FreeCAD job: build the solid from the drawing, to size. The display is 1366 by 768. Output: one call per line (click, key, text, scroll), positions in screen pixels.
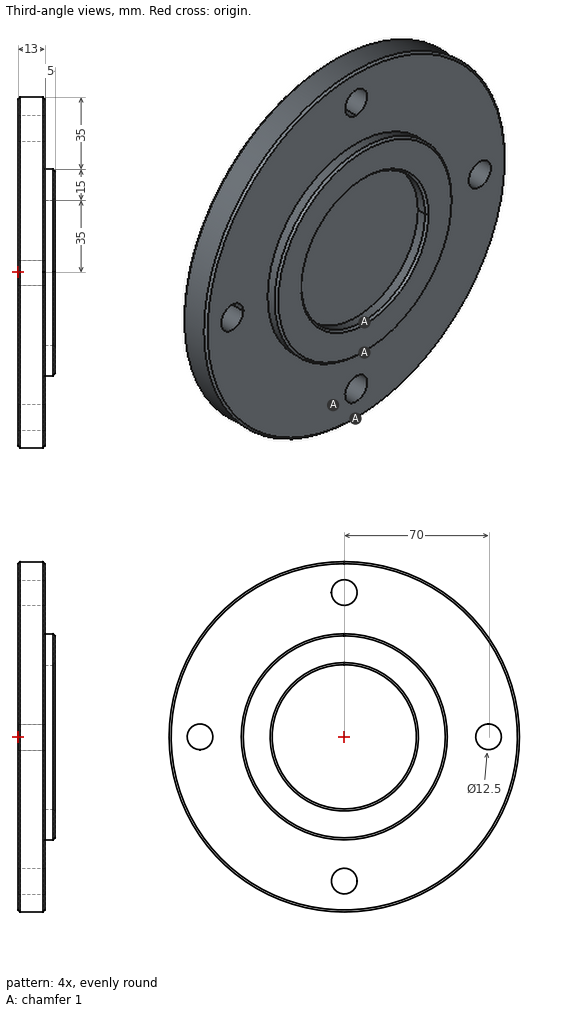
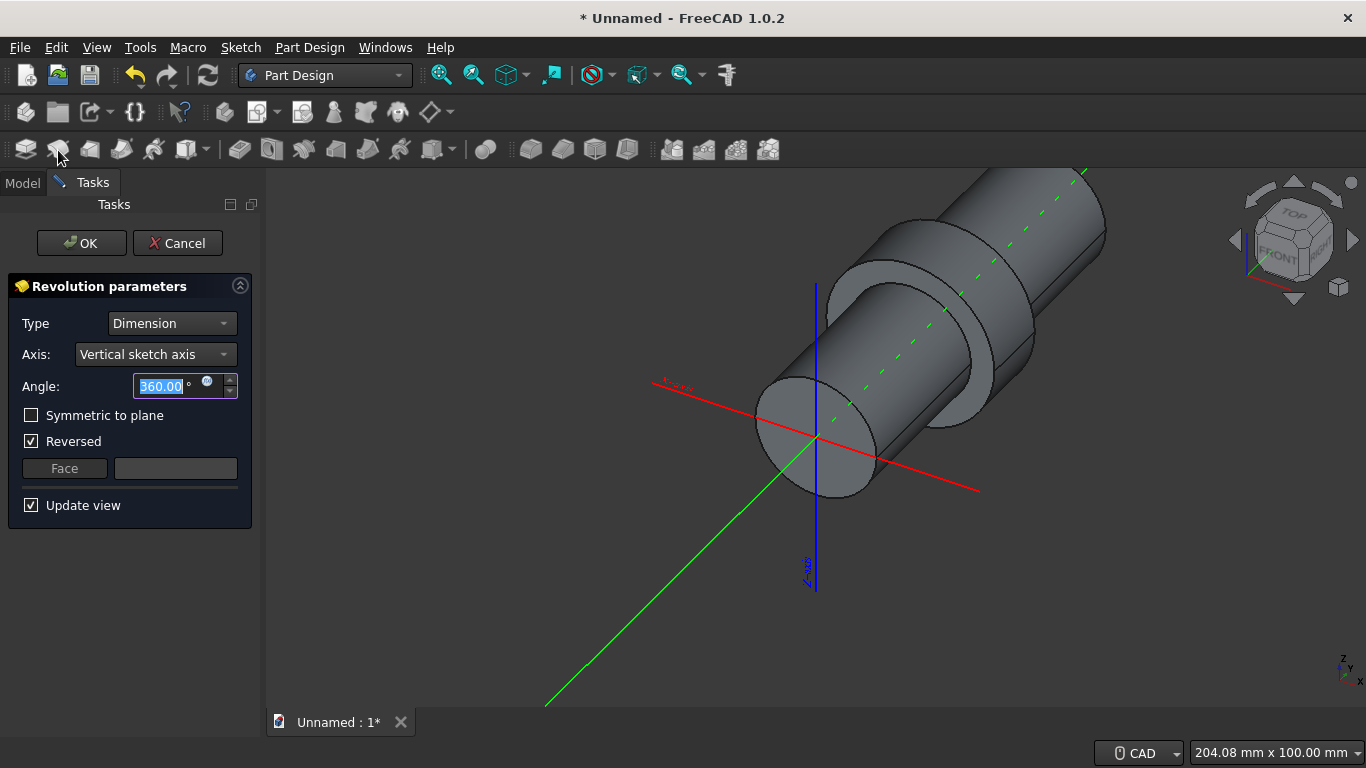
click(156, 354)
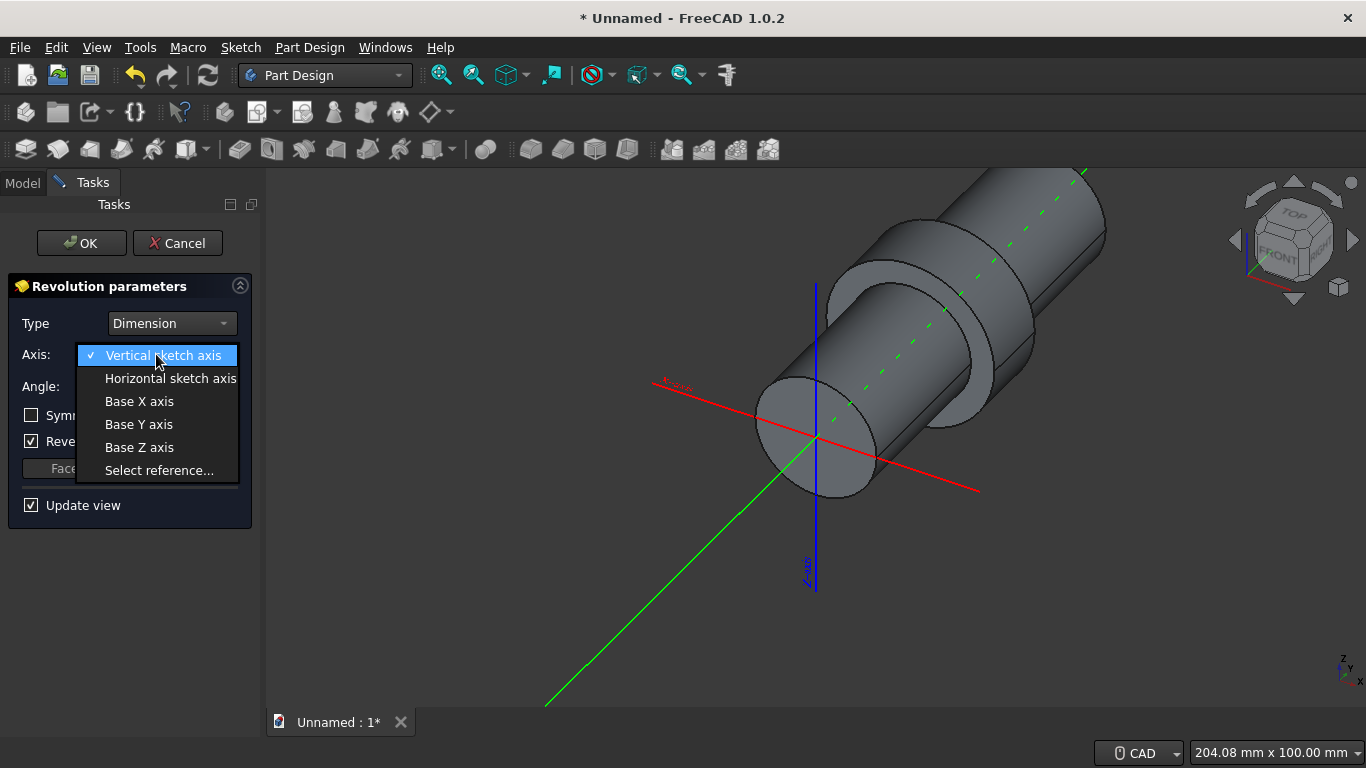
click(156, 378)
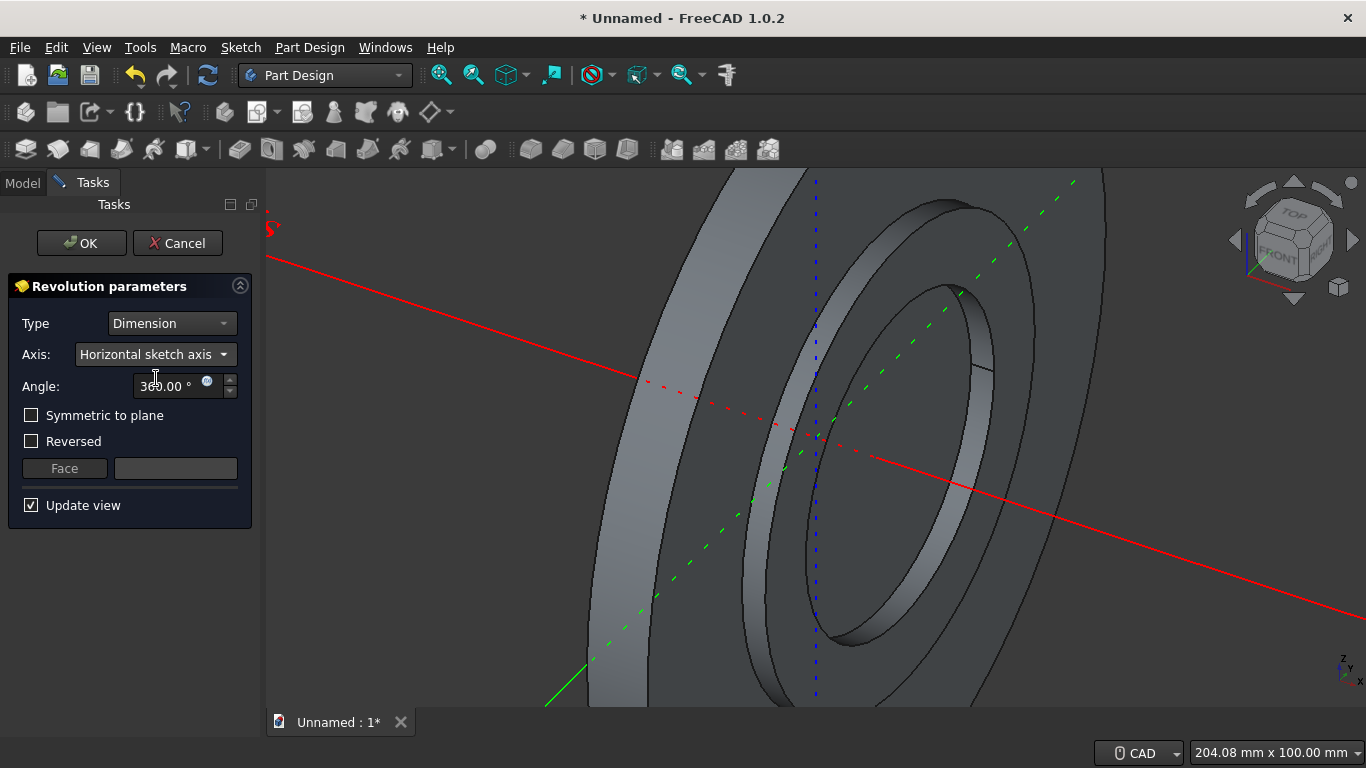
click(82, 243)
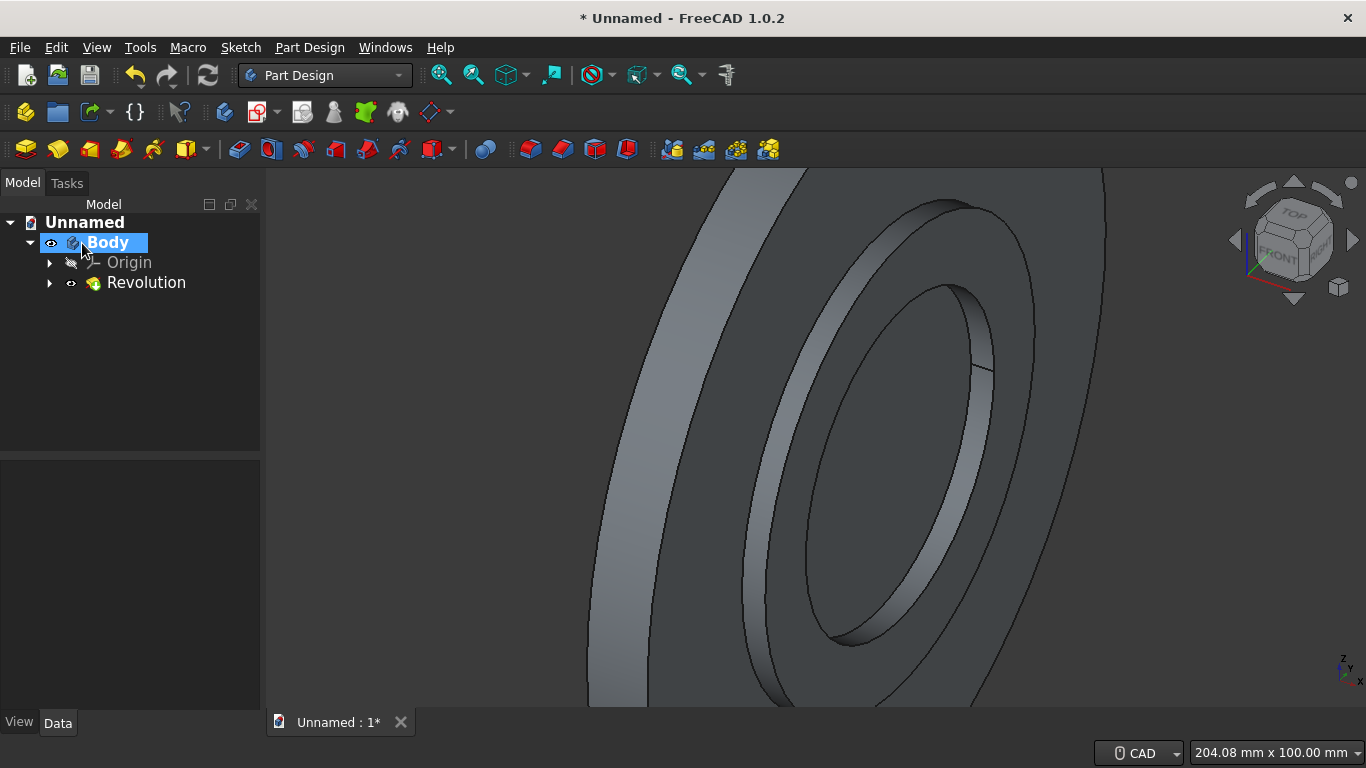
click(442, 76)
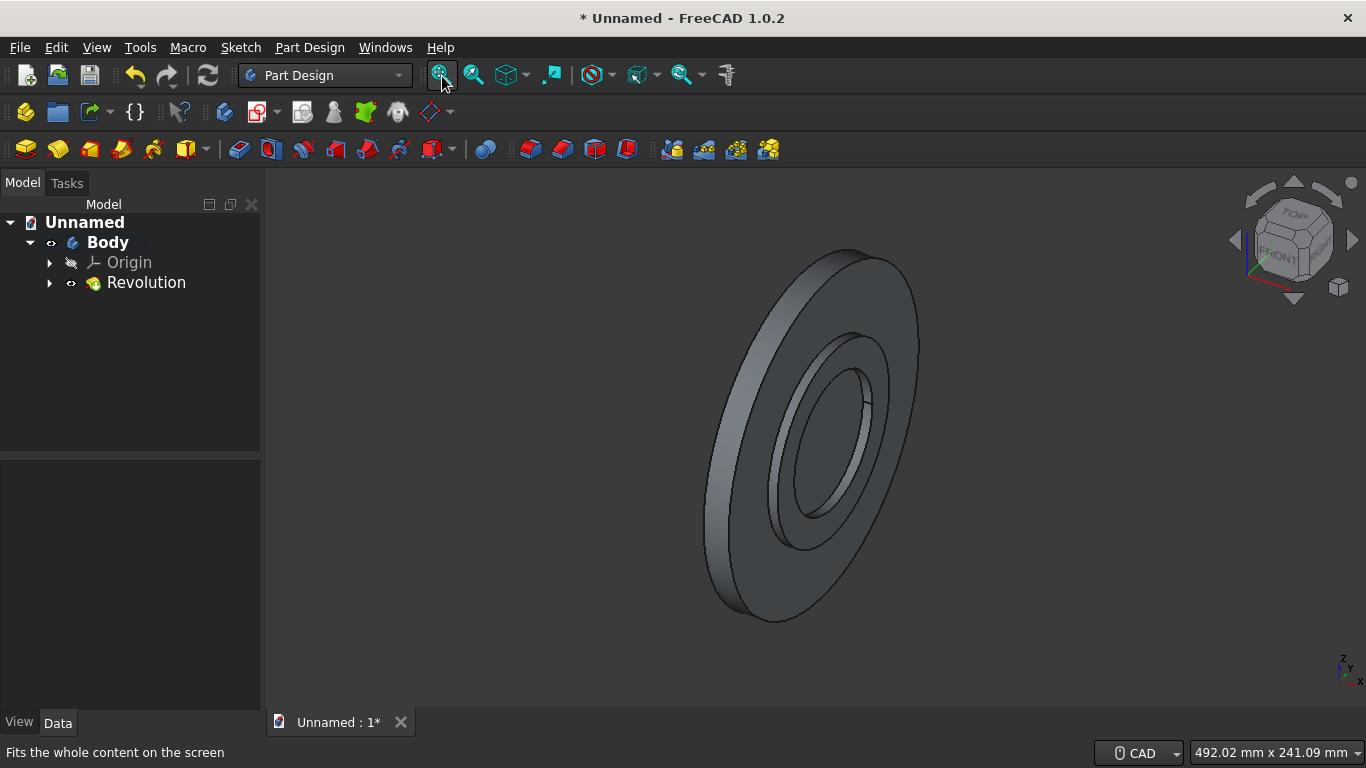
key(6)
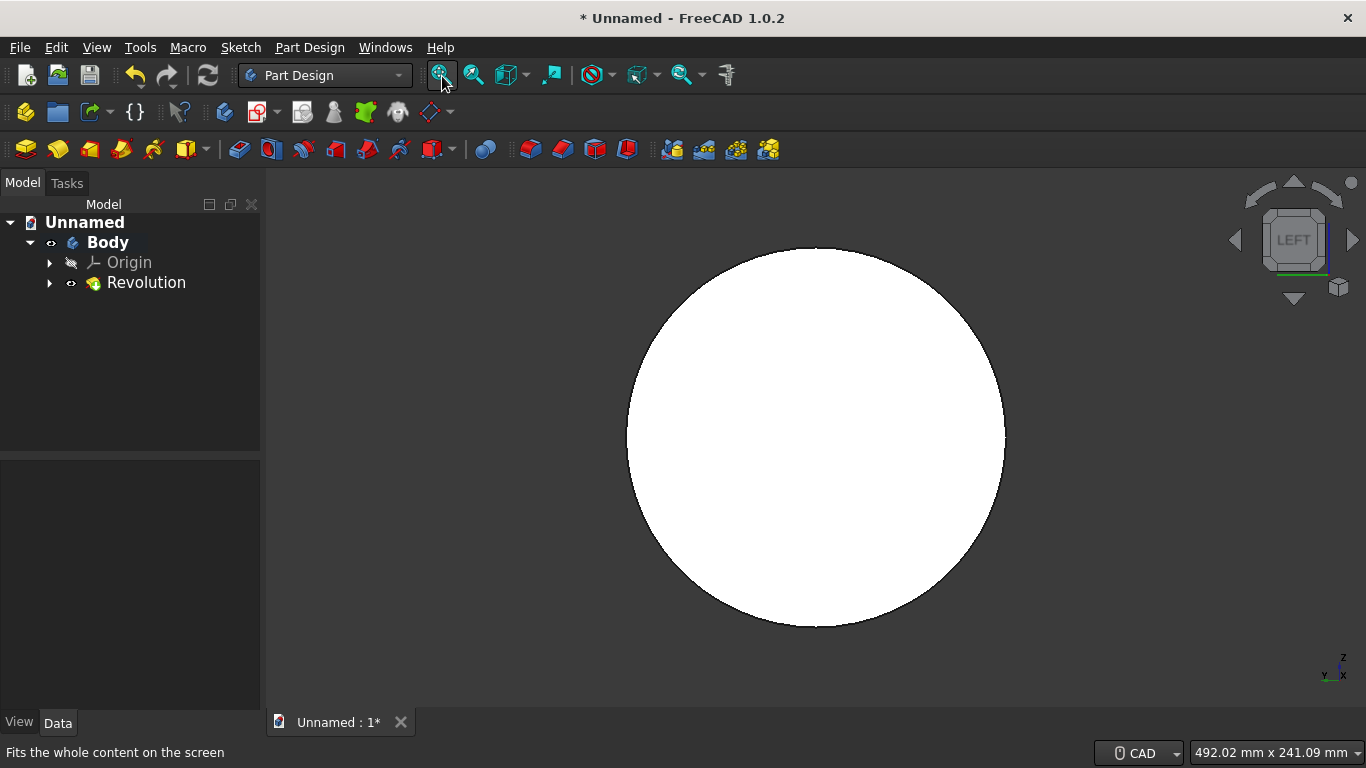
click(816, 436)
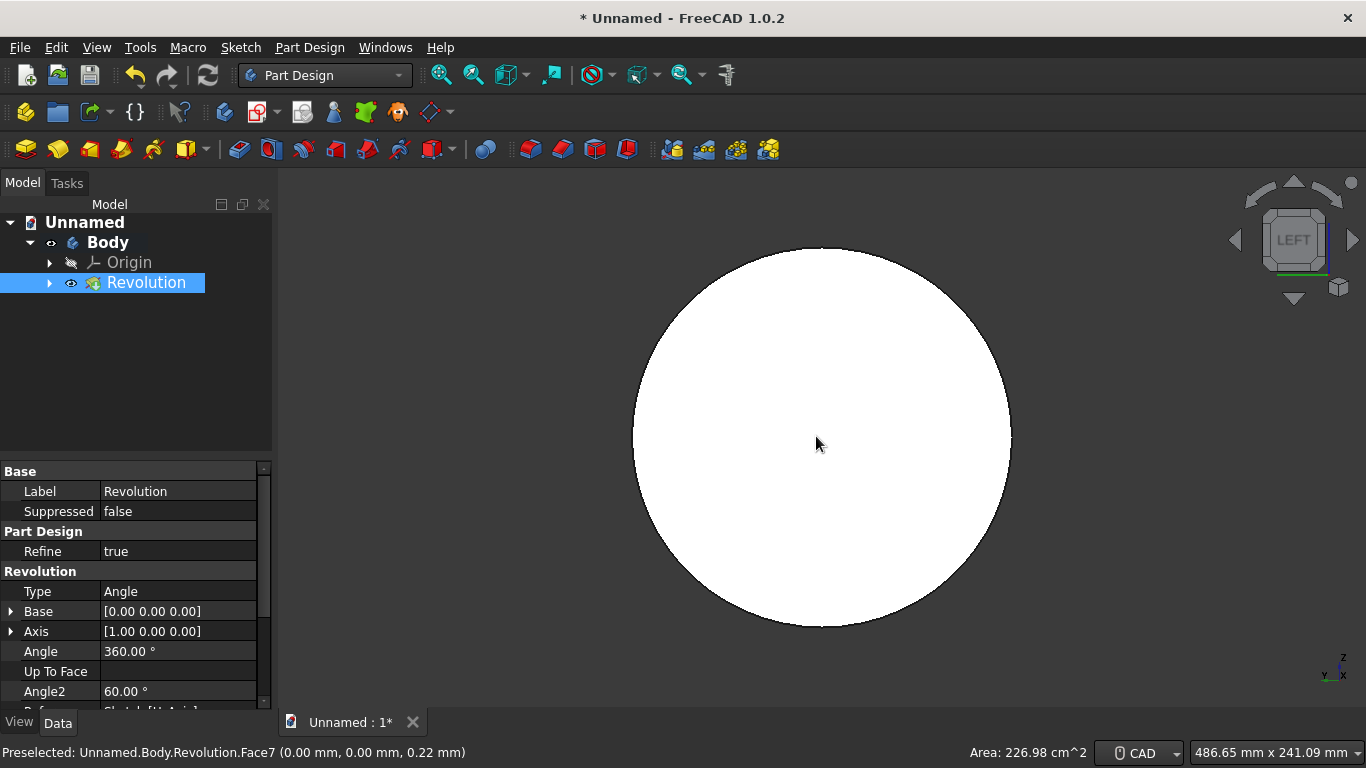
click(258, 112)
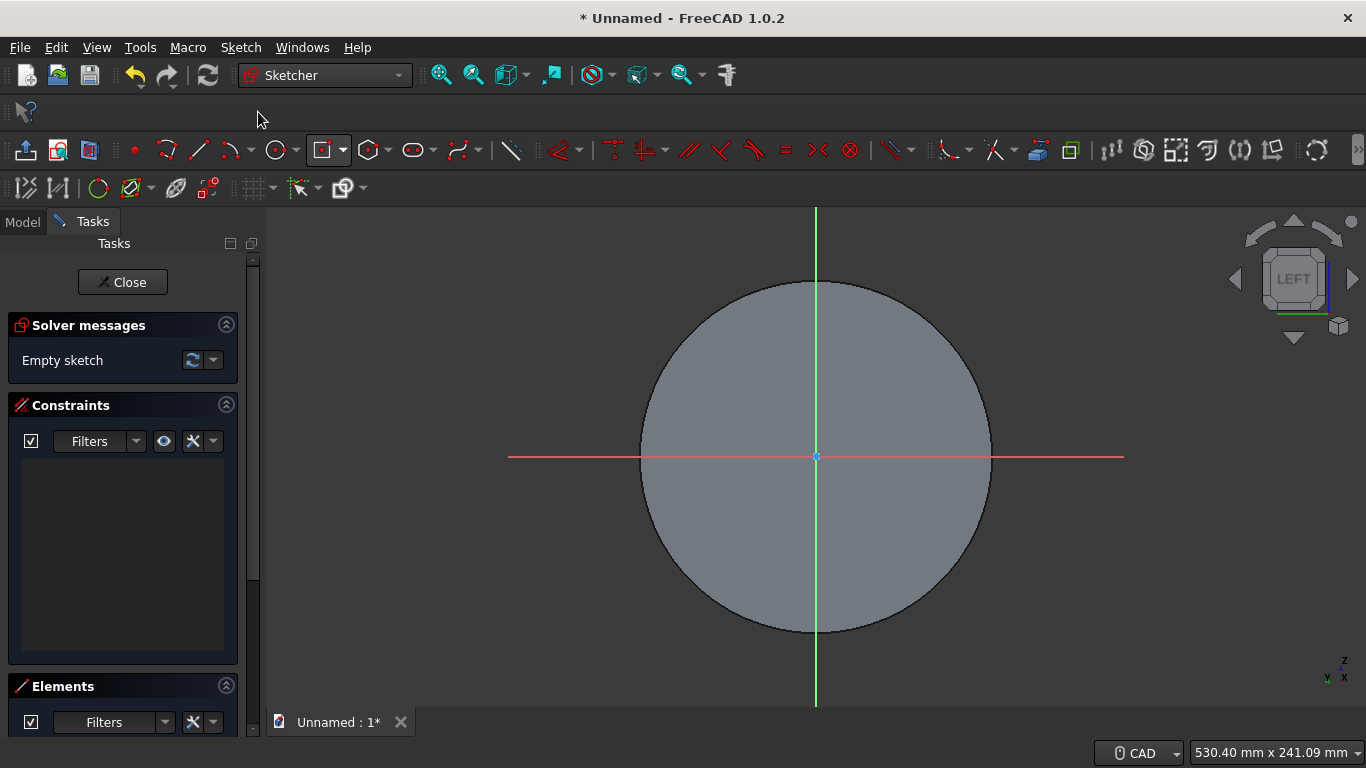
scroll(663, 457, up, 12)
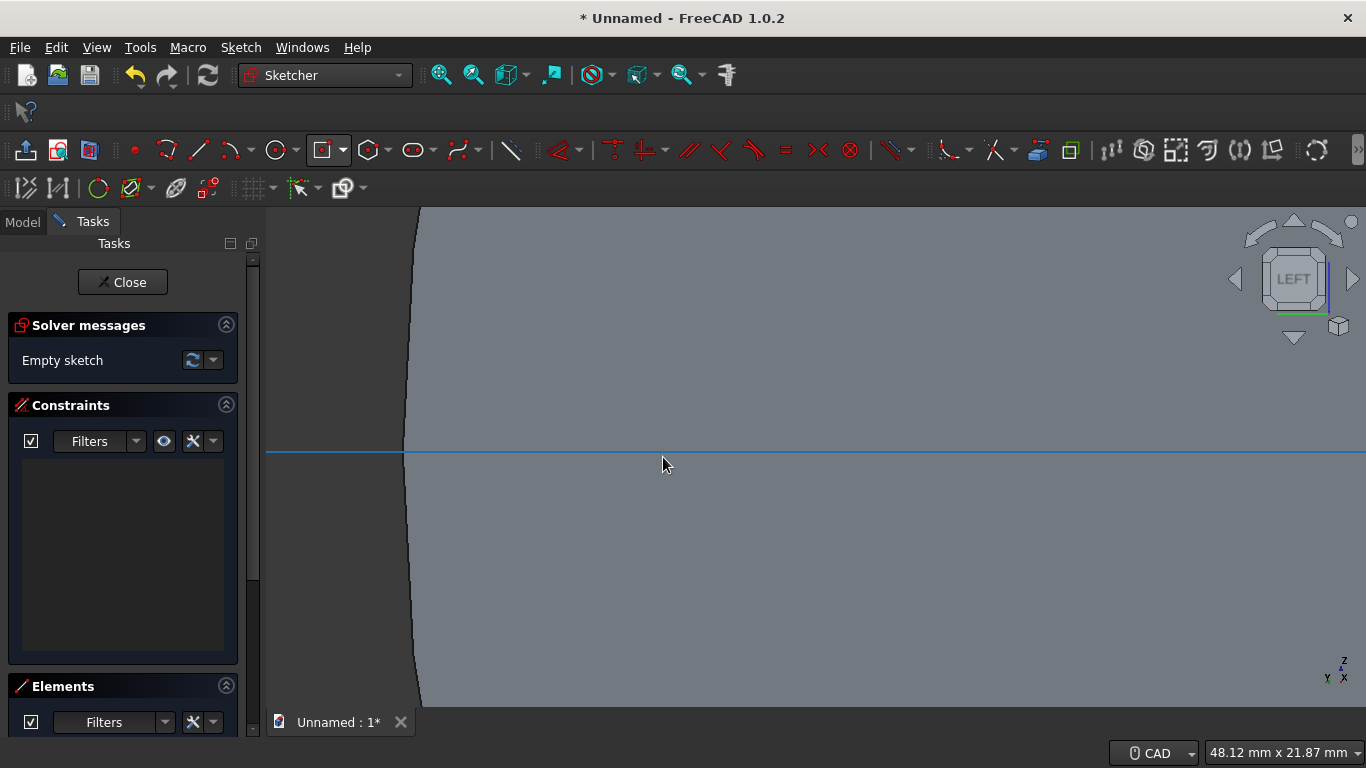
click(276, 150)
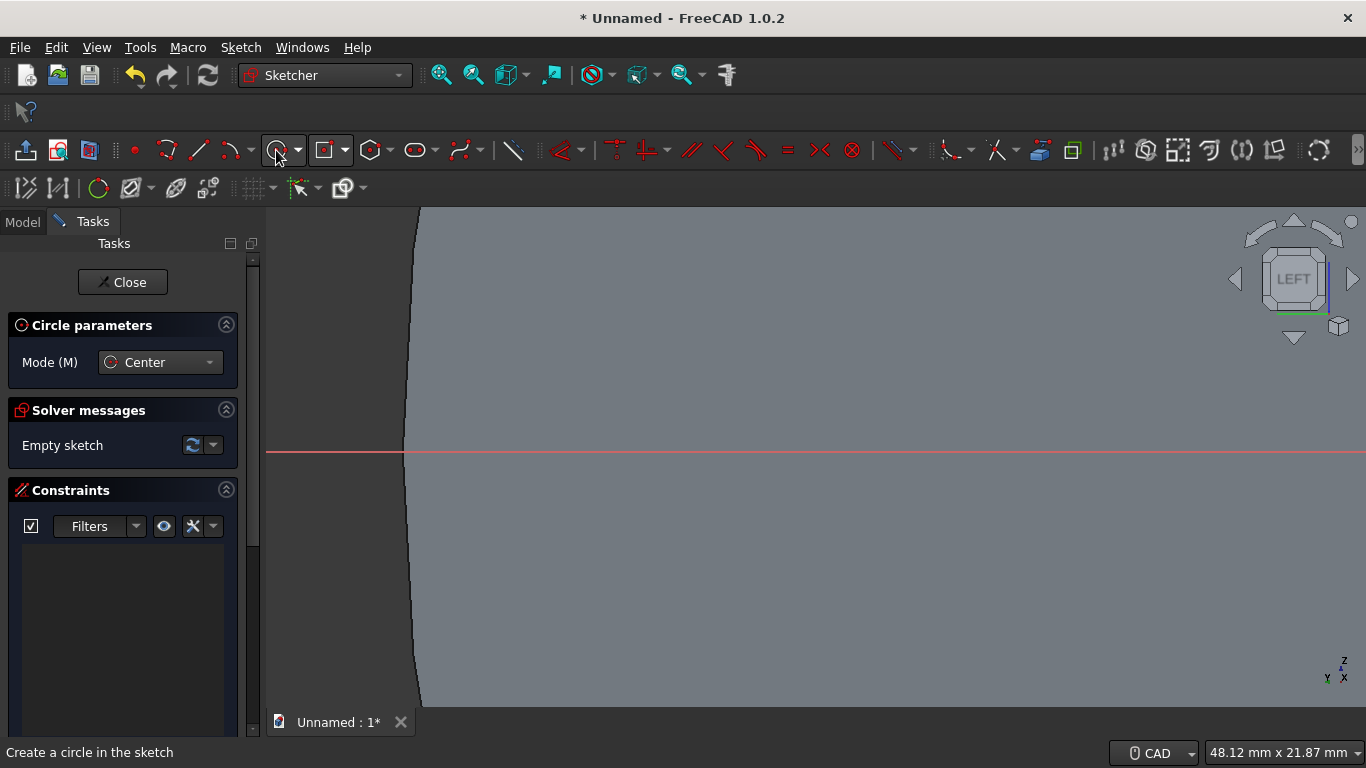
click(746, 452)
move(847, 351)